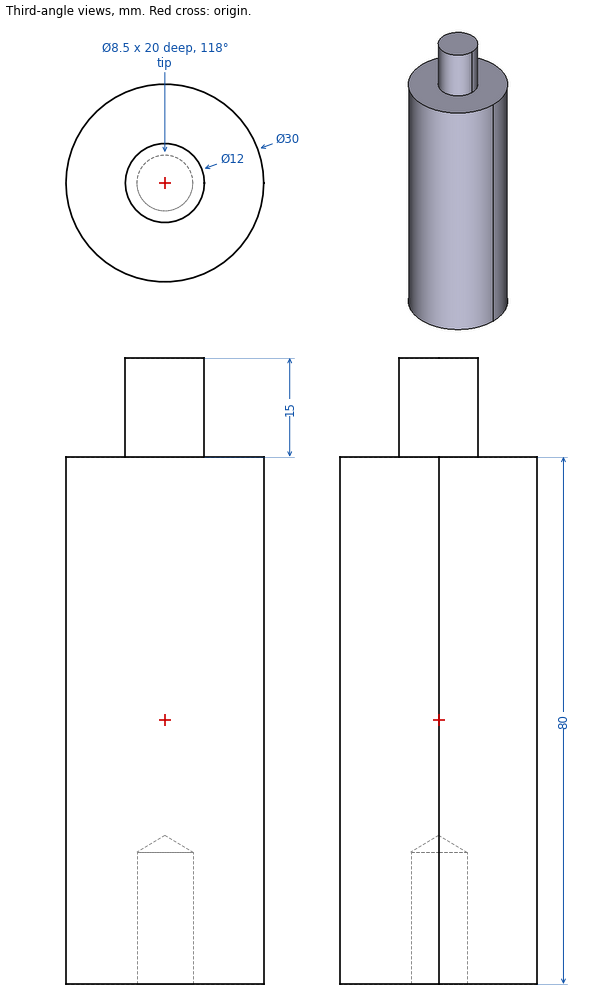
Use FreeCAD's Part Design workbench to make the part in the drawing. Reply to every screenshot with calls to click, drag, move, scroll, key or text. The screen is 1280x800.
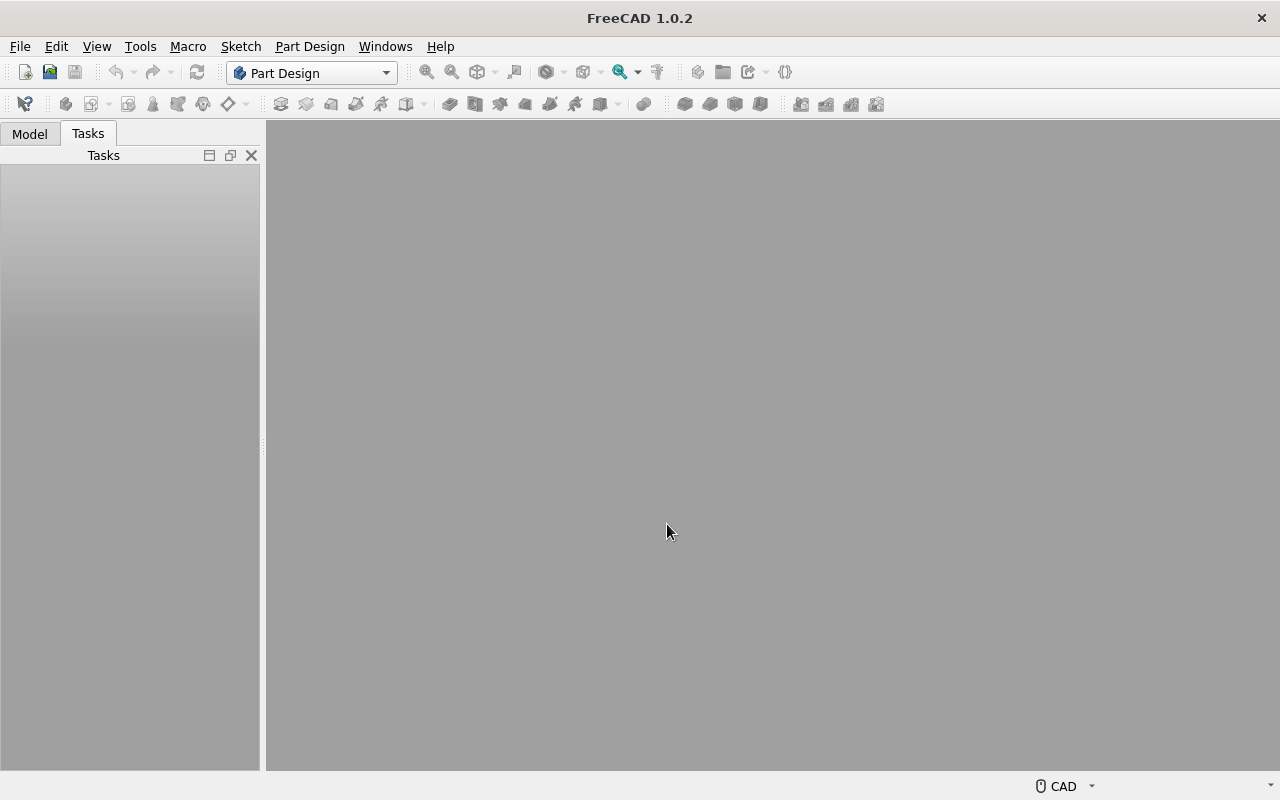
click(25, 72)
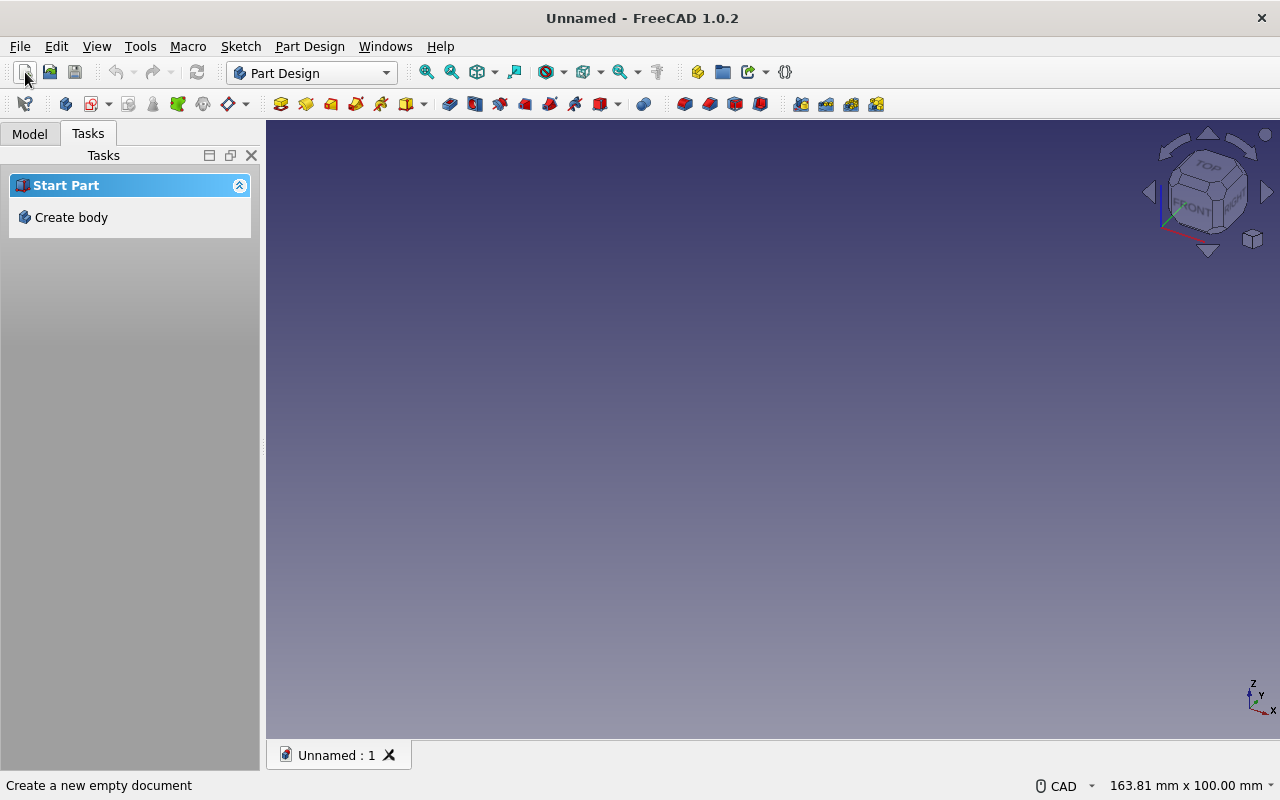
click(90, 104)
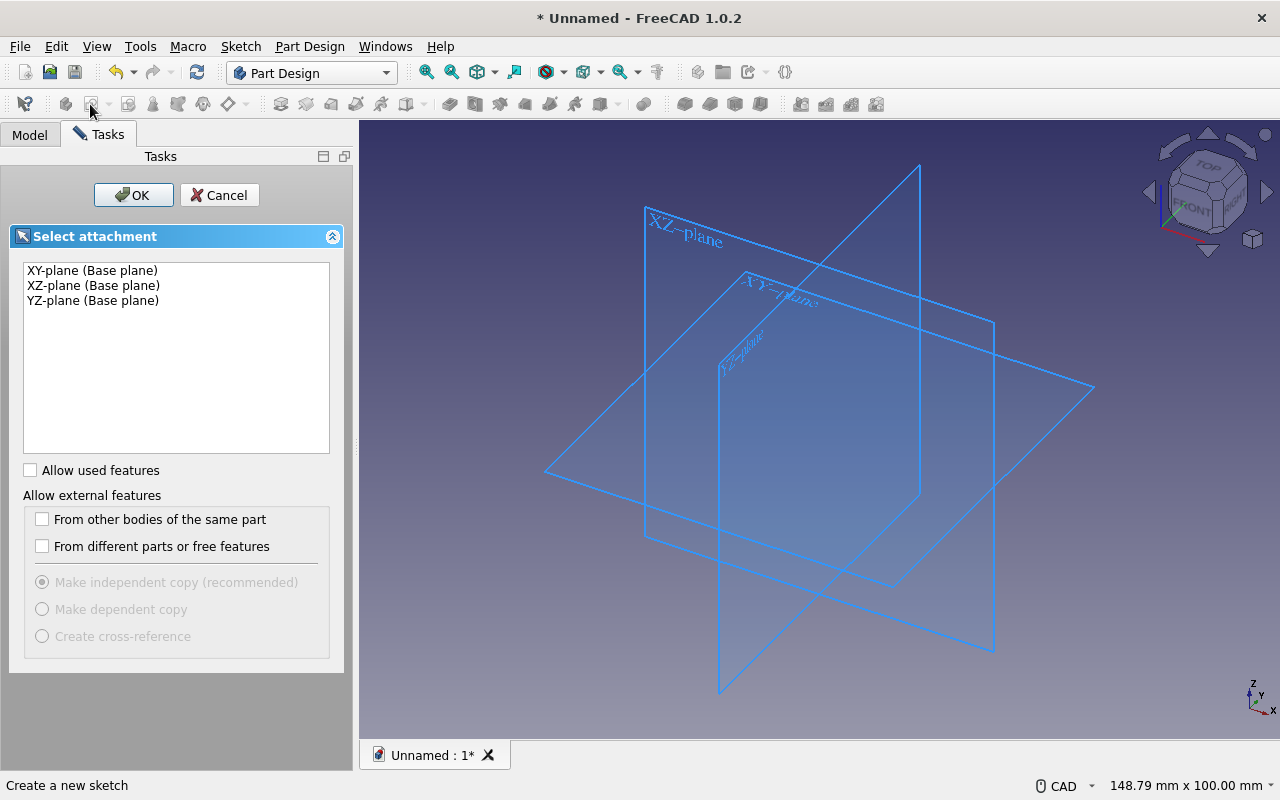
click(84, 270)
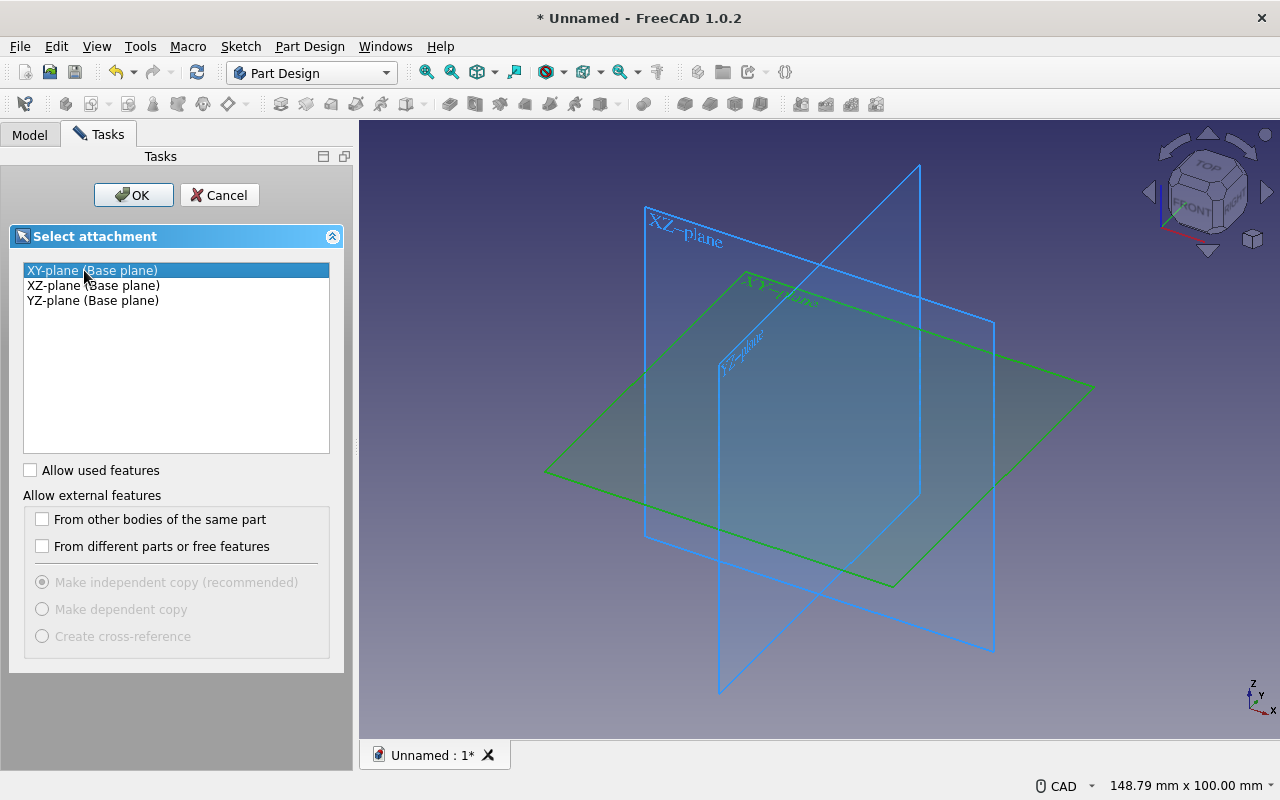
click(134, 195)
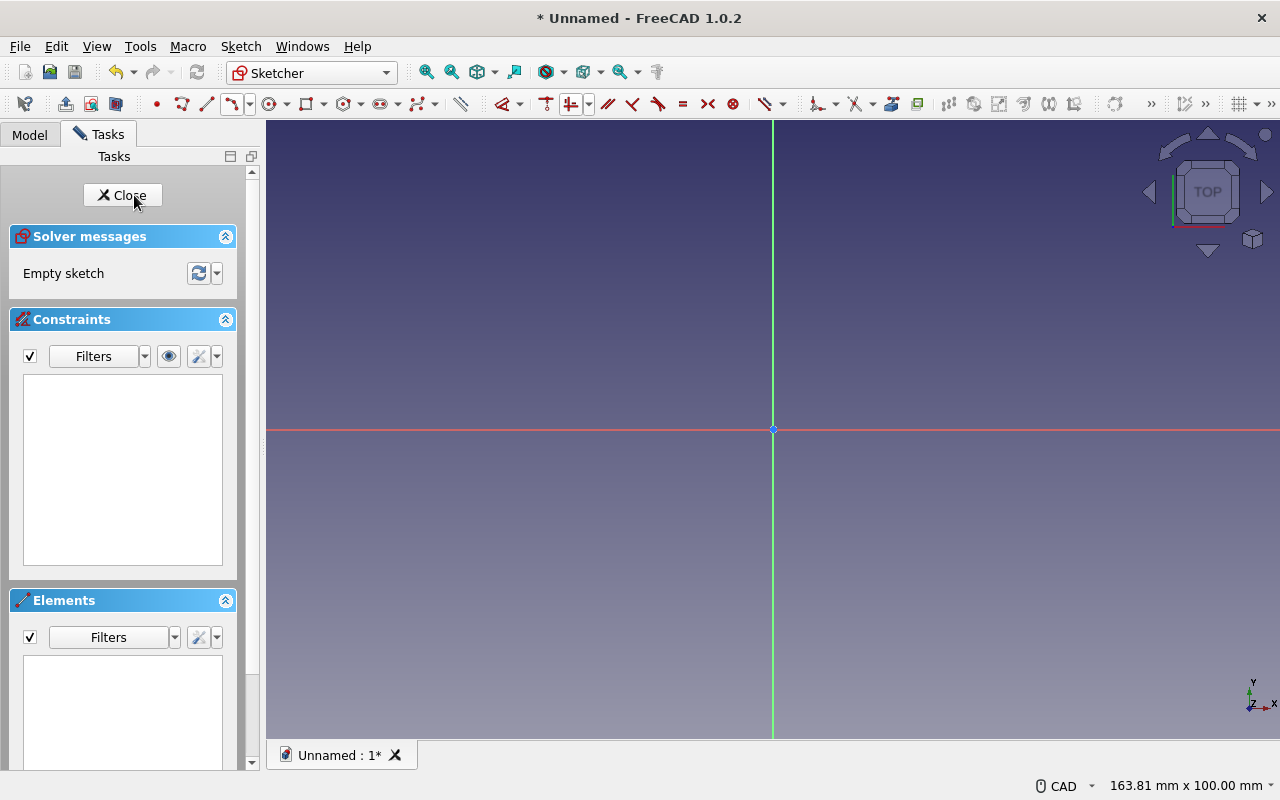
scroll(829, 430, up, 4)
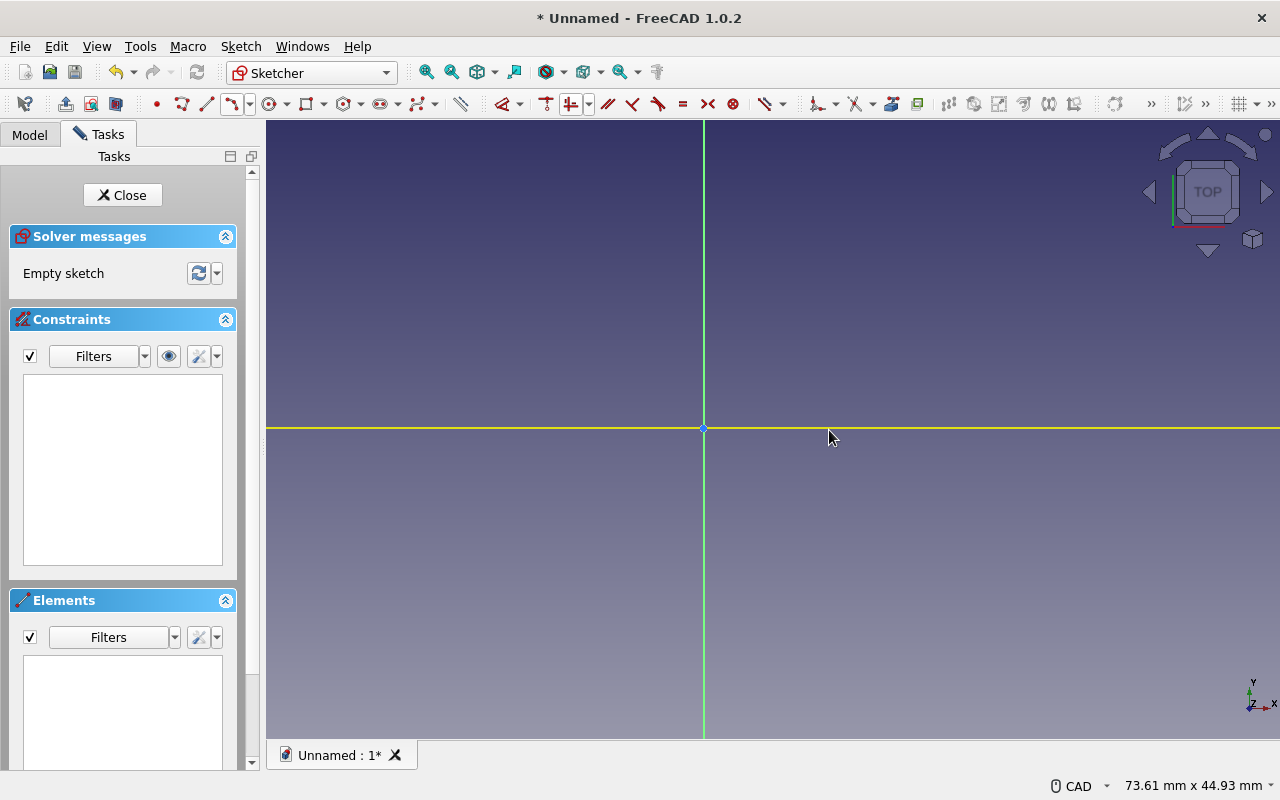
click(268, 104)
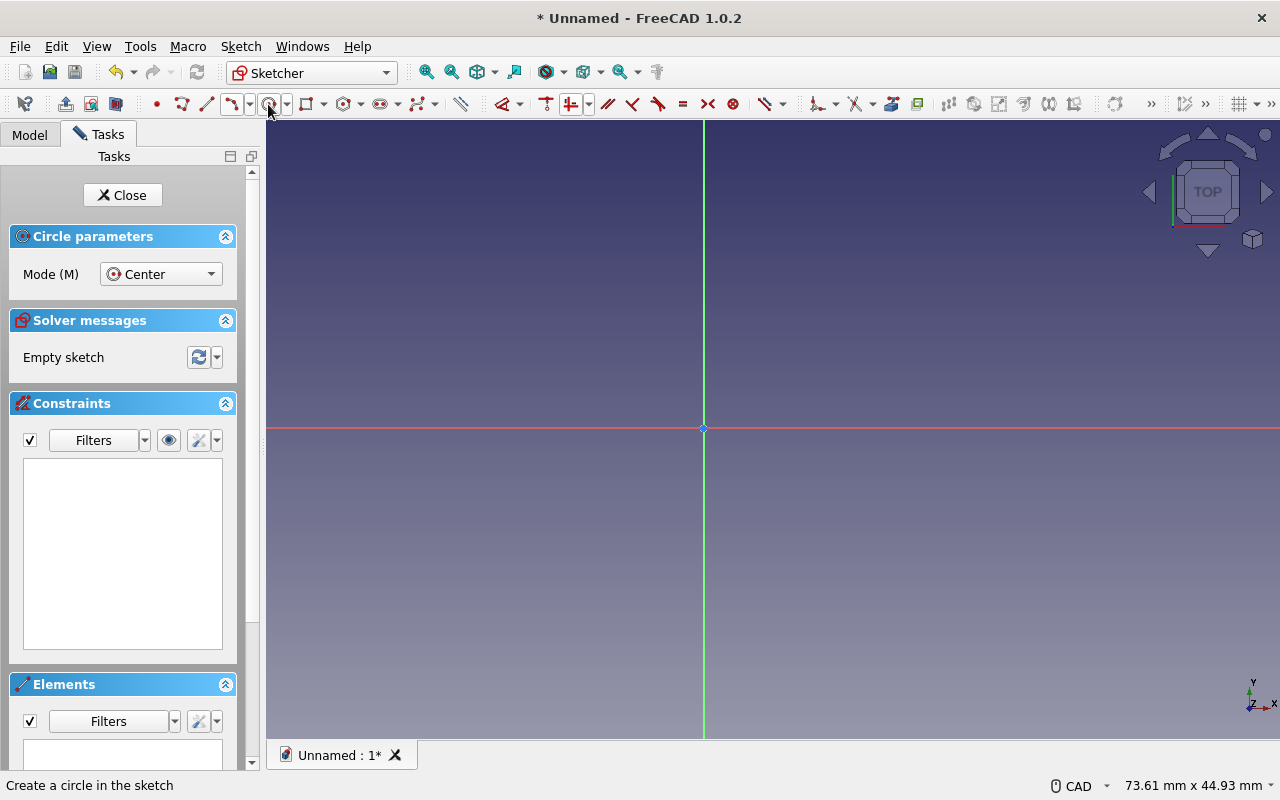
click(704, 428)
move(850, 282)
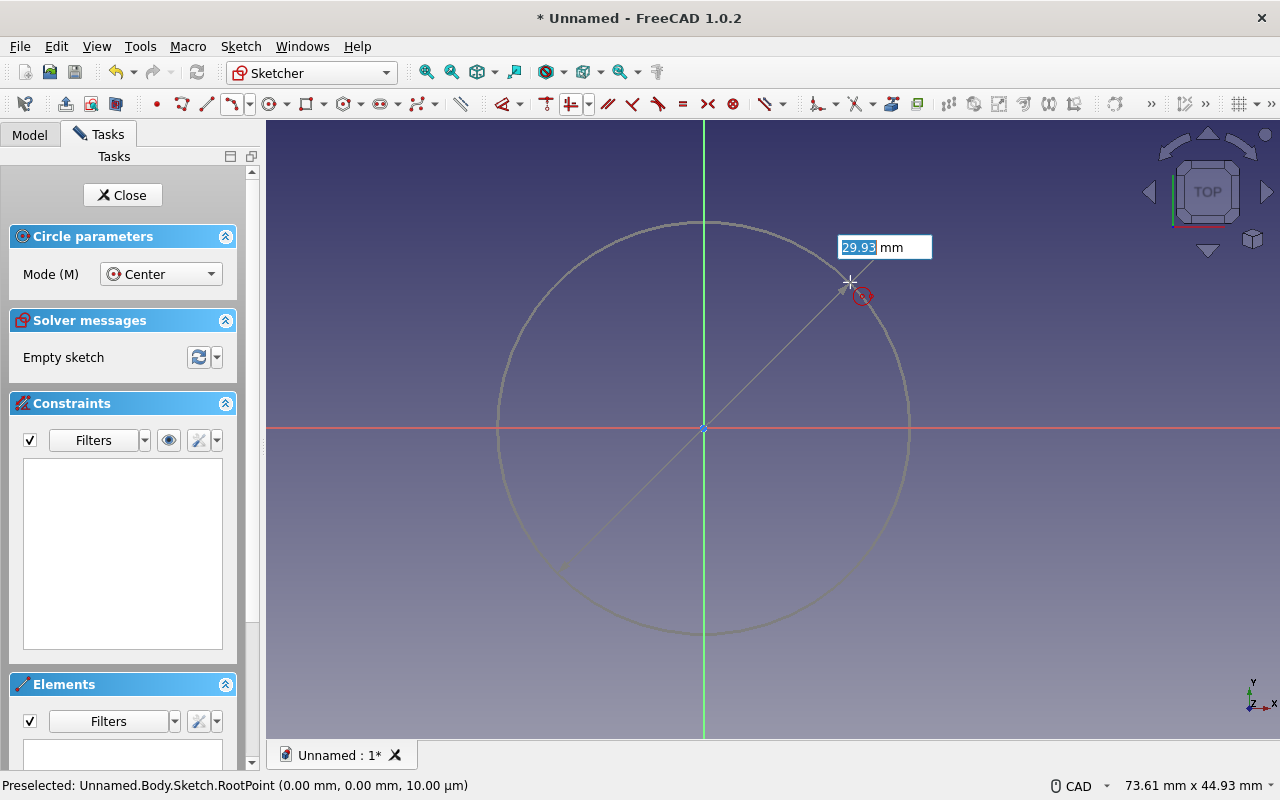
text(30)
key(Return)
key(Escape)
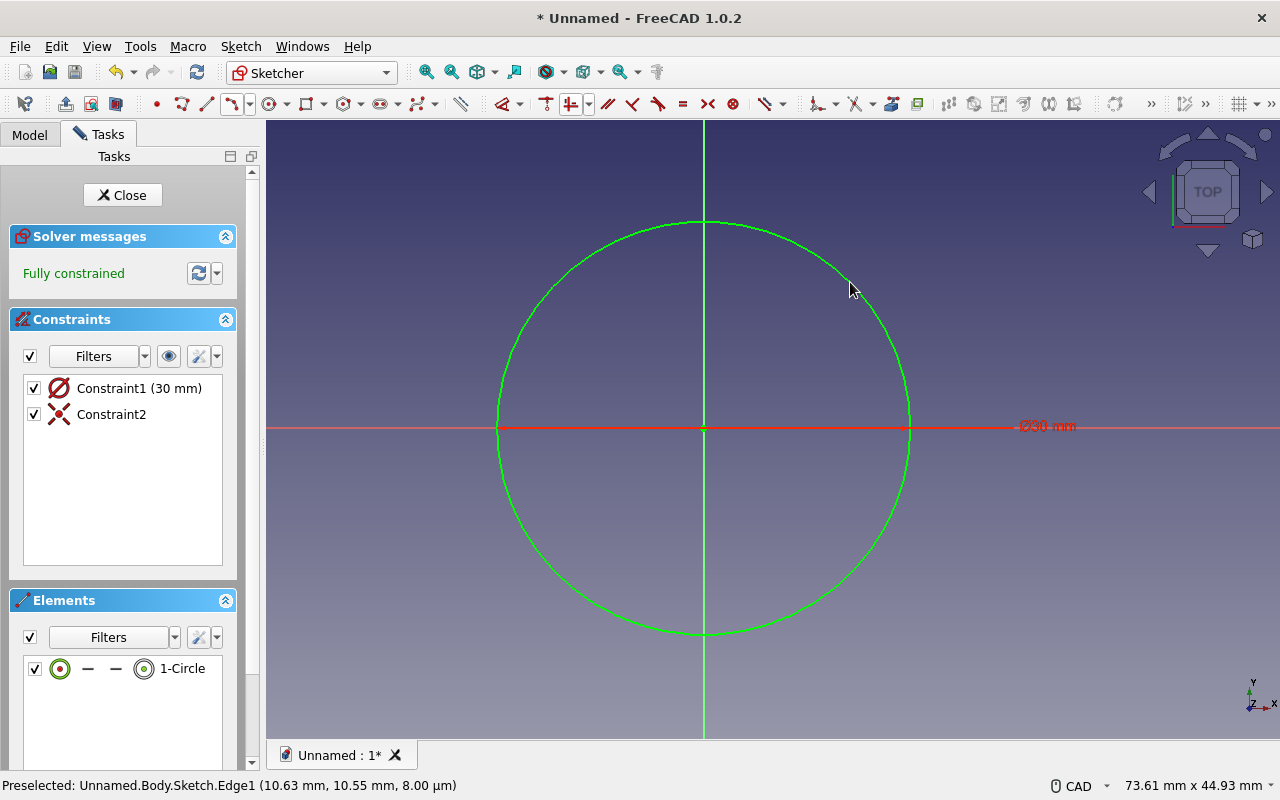
click(123, 195)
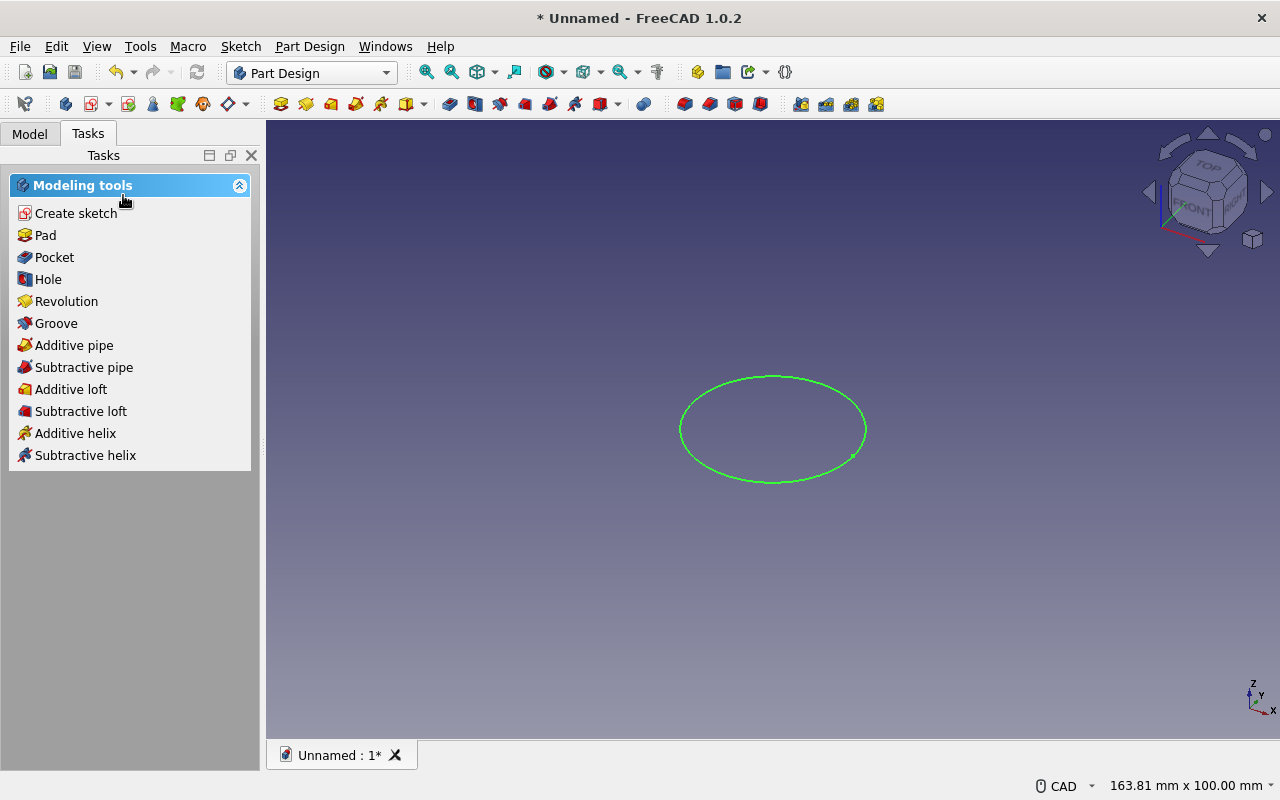
click(281, 104)